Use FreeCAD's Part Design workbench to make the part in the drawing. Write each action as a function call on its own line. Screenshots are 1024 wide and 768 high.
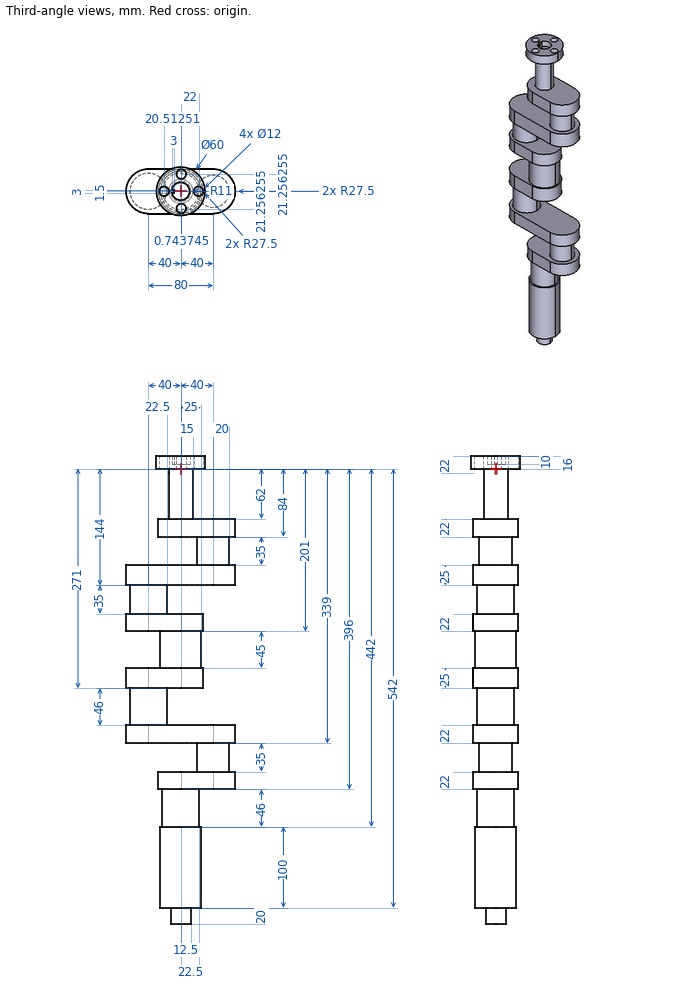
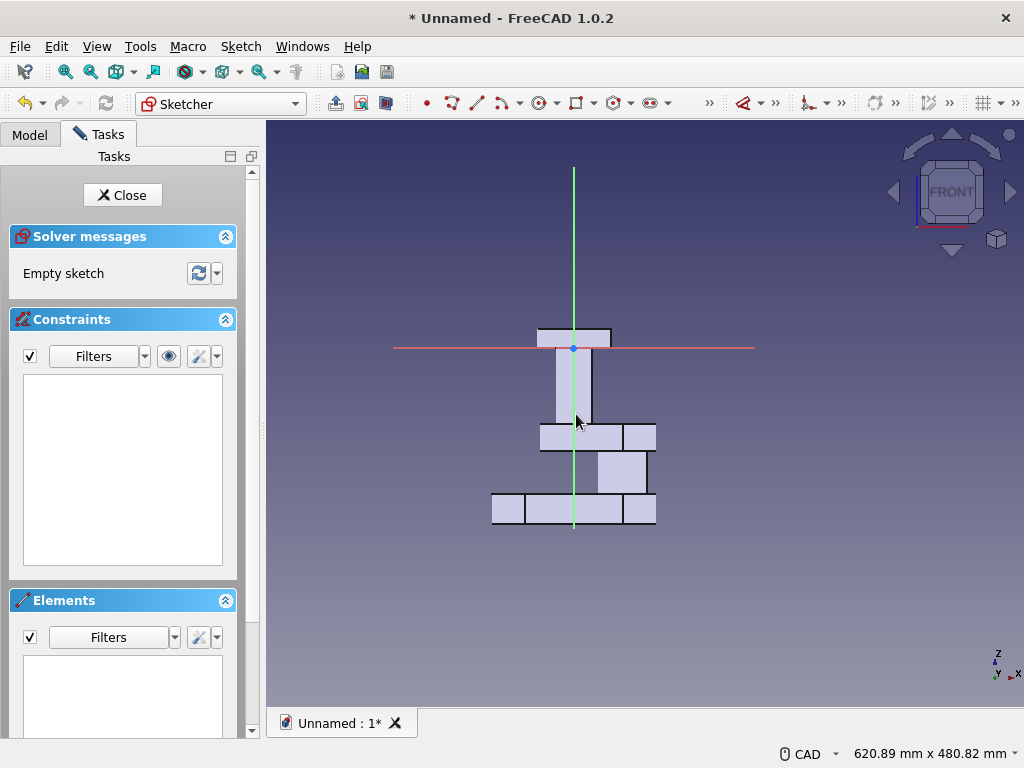
scroll(531, 582, up, 9)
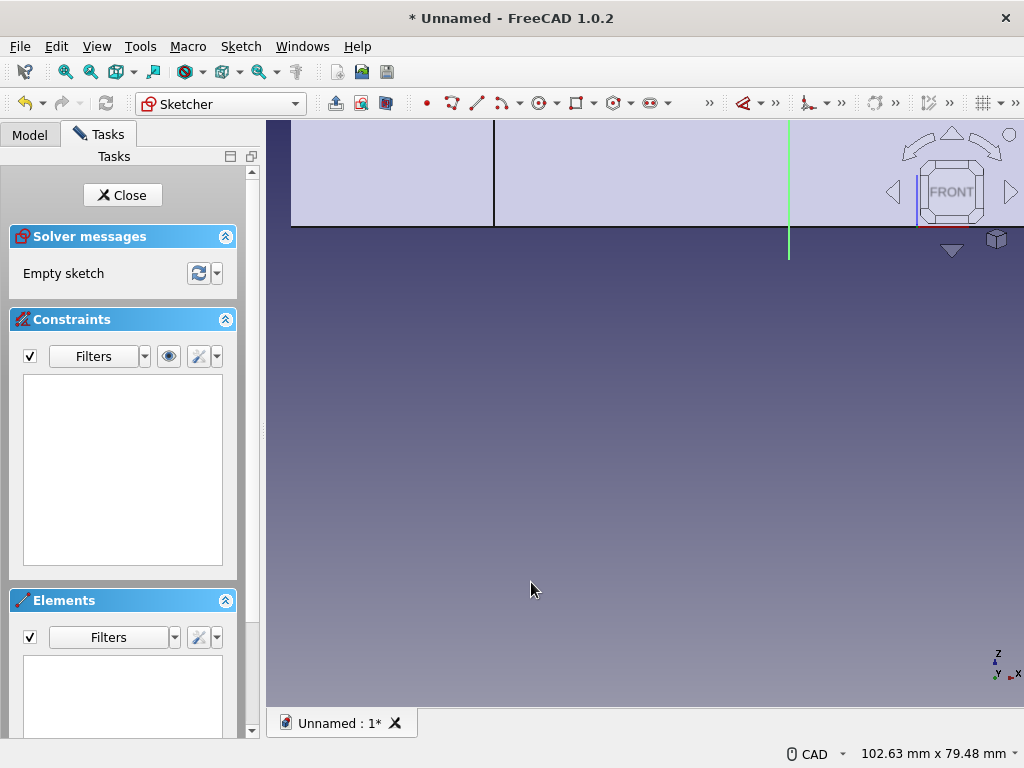
click(576, 104)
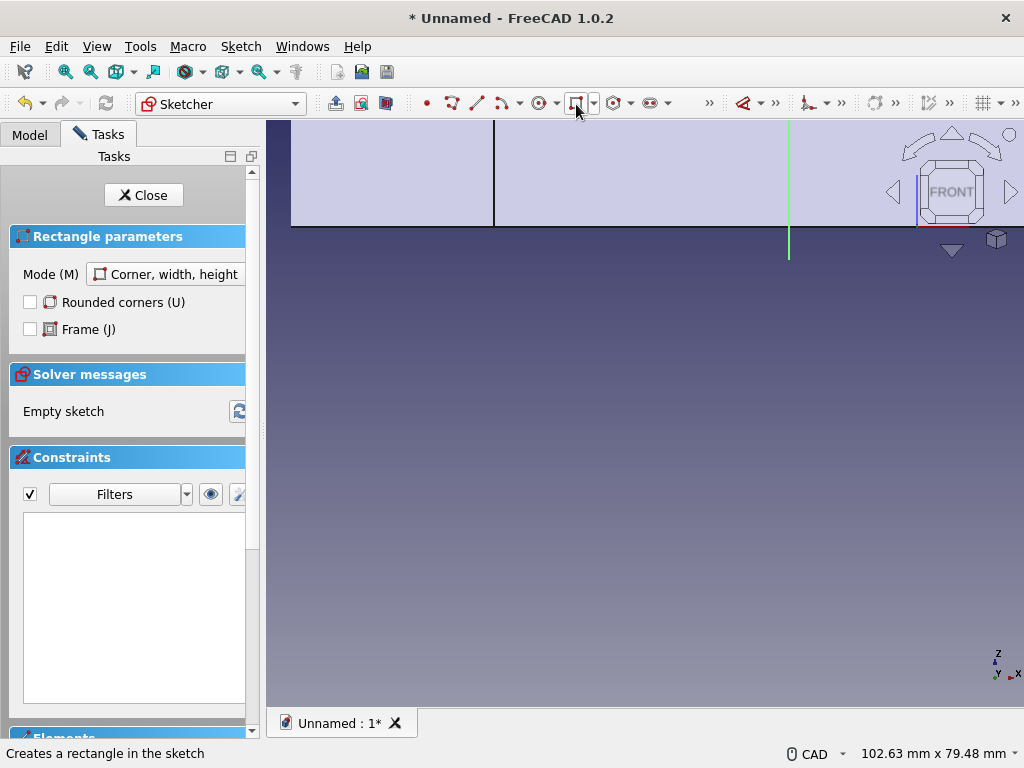
click(494, 227)
move(660, 486)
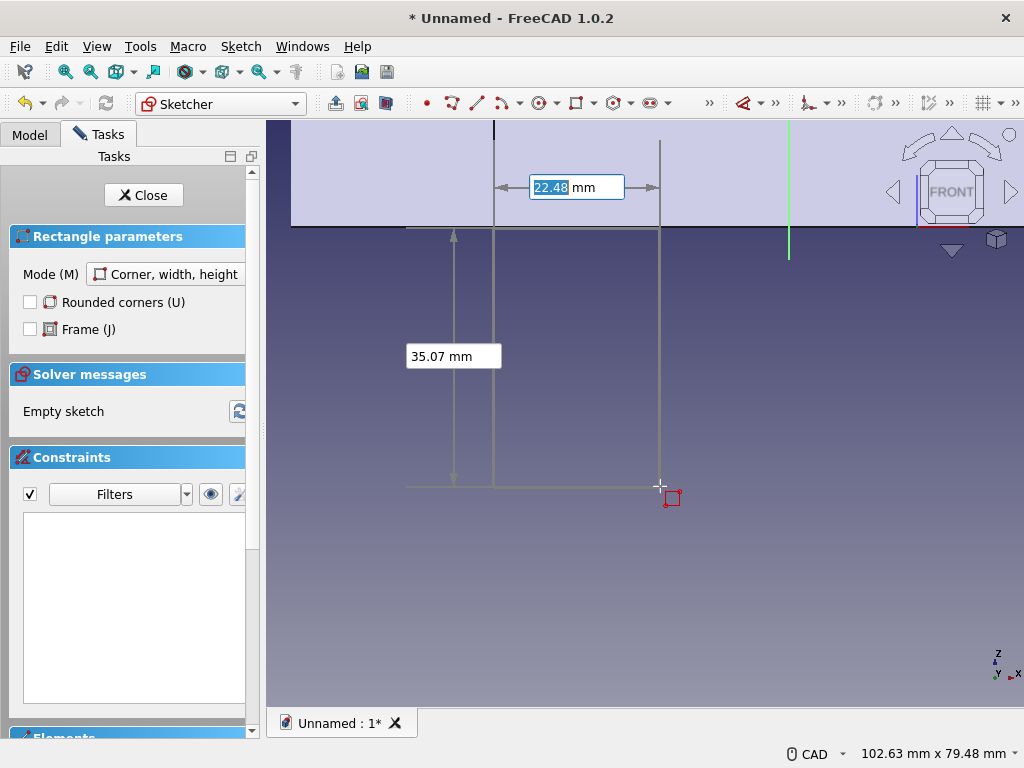
text(22.5)
key(Tab)
text(35)
key(Return)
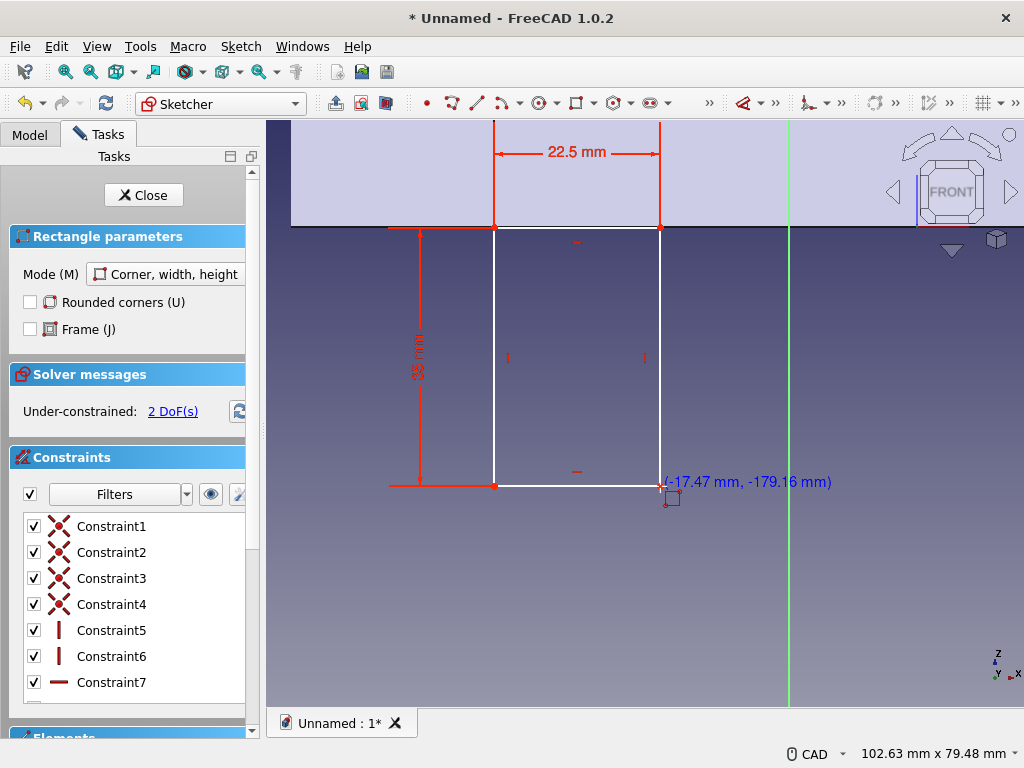
key(g)
key(l)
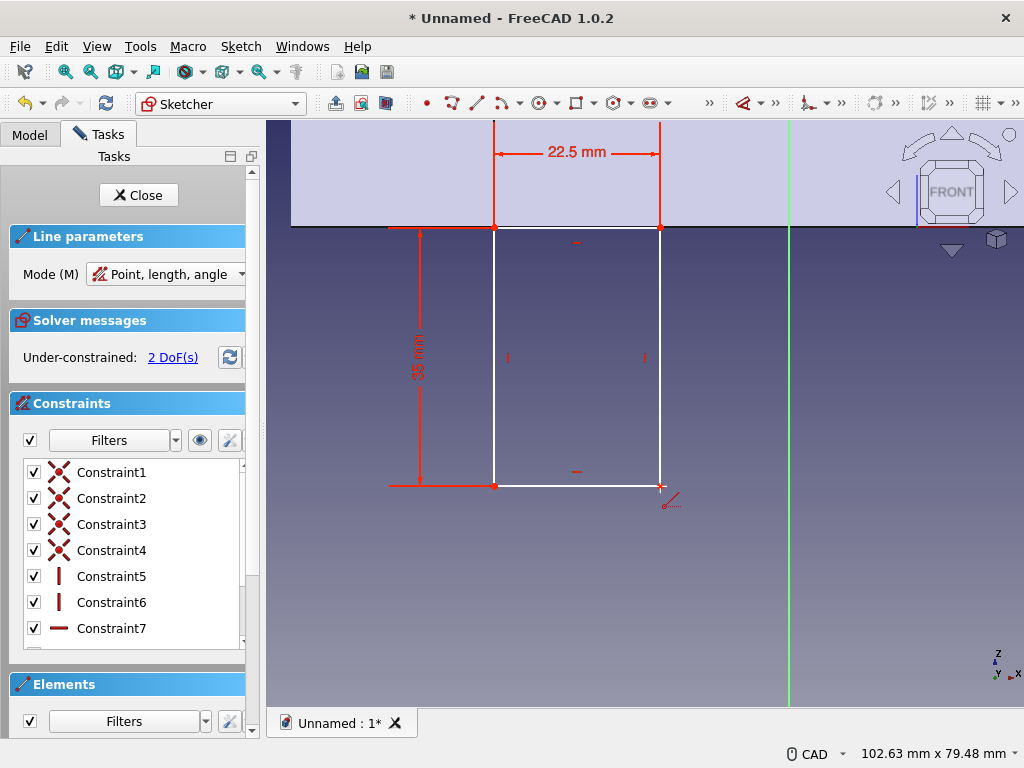
click(494, 512)
click(494, 589)
key(Escape)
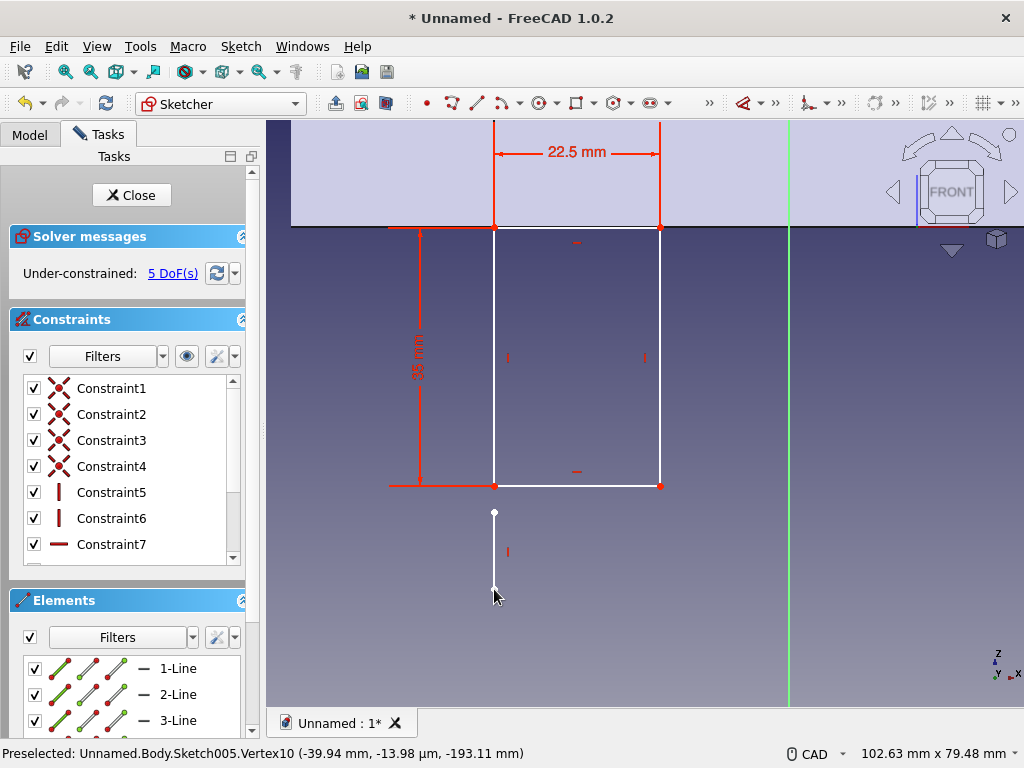
click(494, 536)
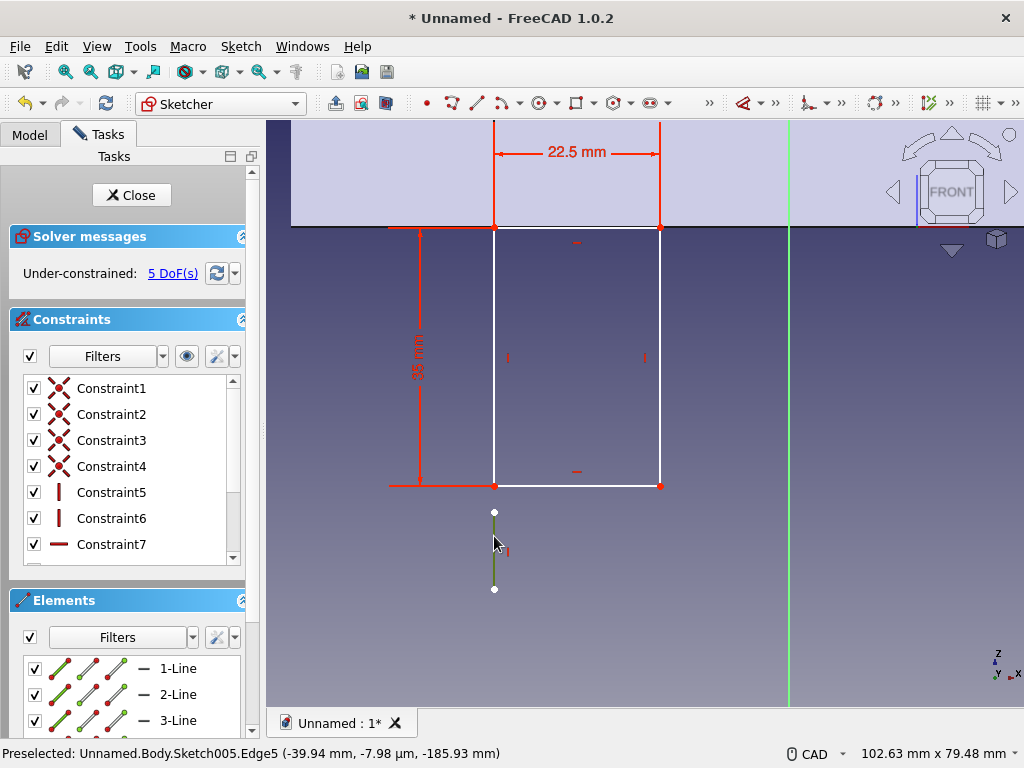
key(g)
key(n)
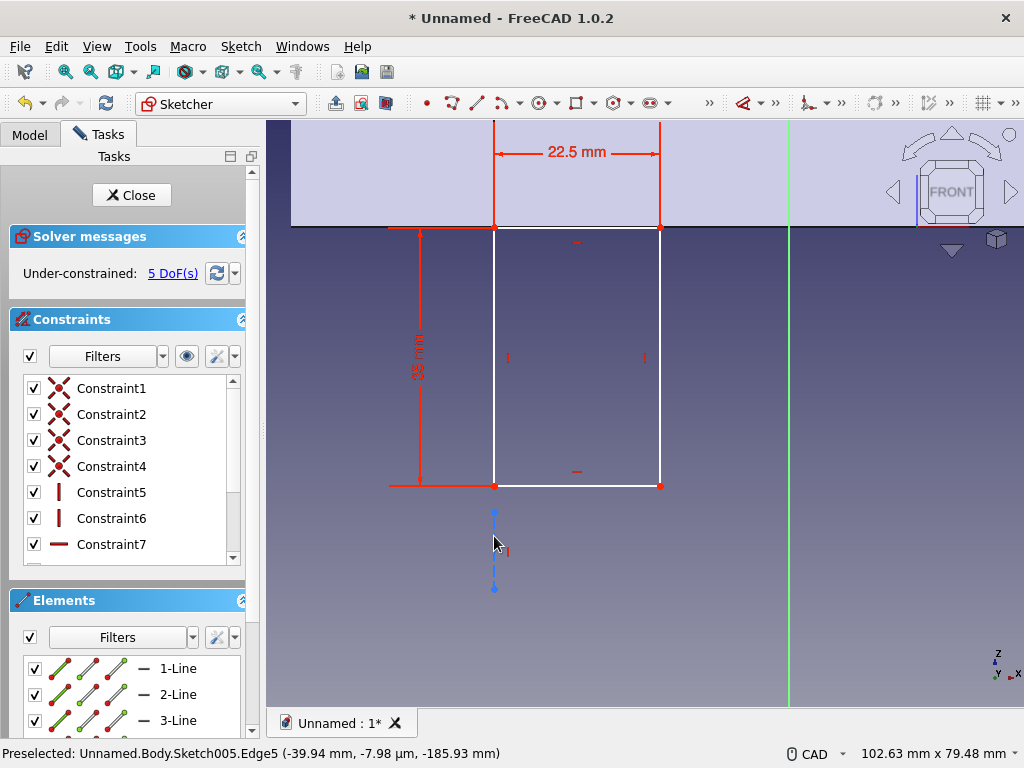
key(d)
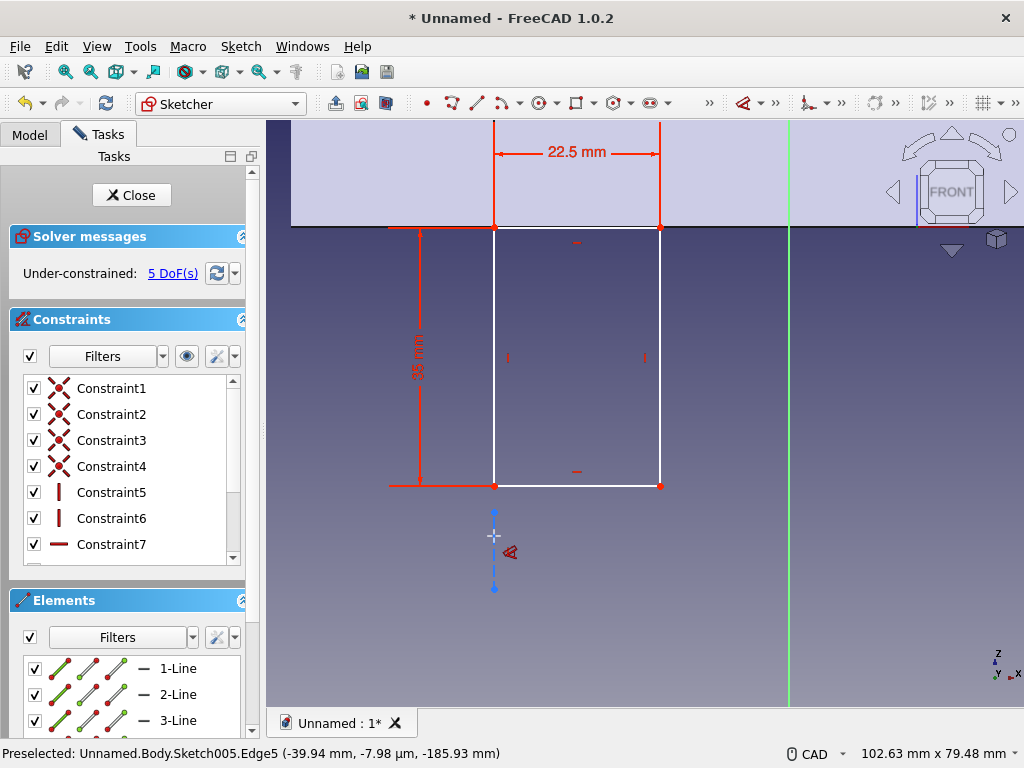
click(494, 228)
click(642, 262)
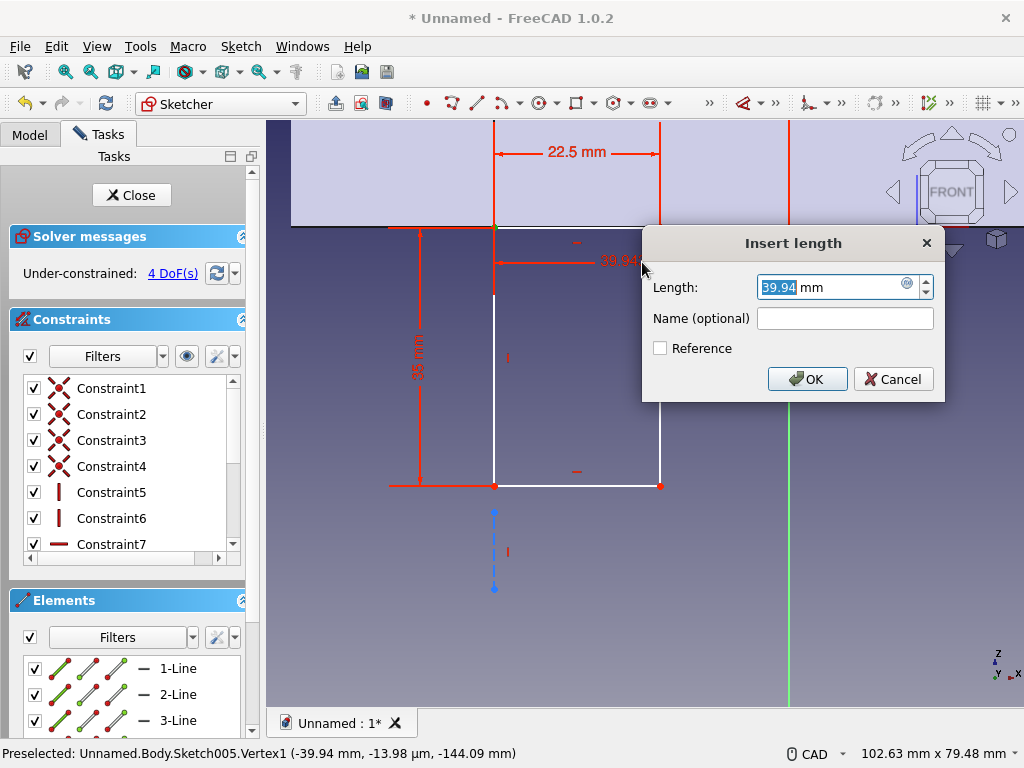
text(40)
key(Return)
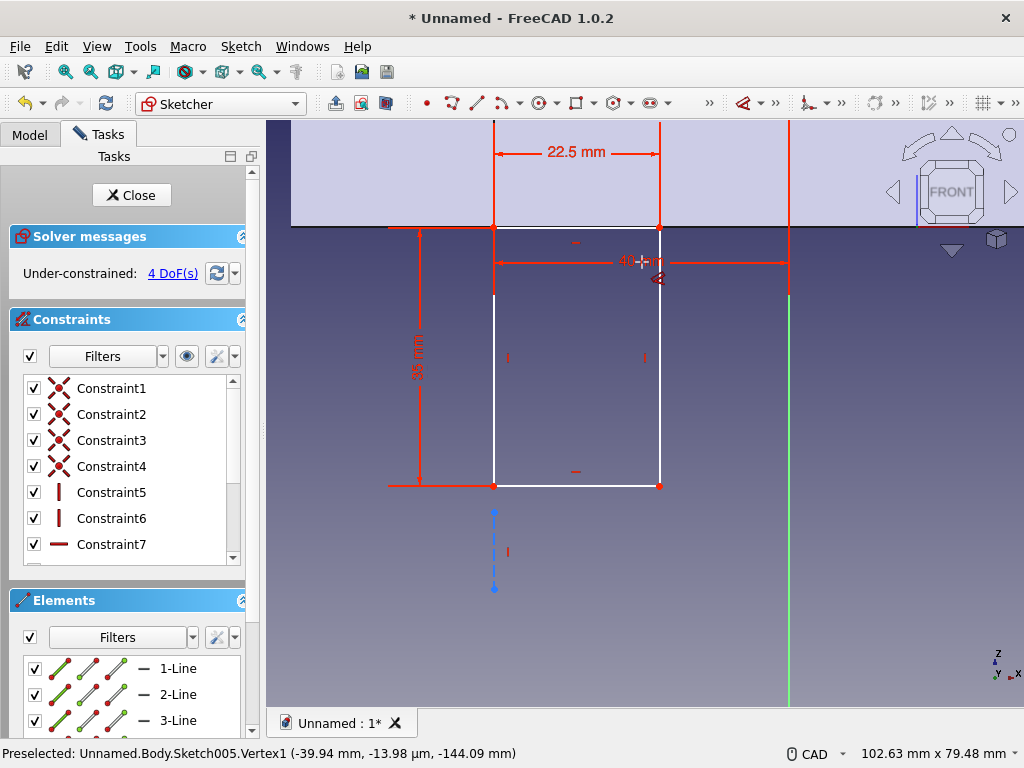
click(494, 513)
click(642, 547)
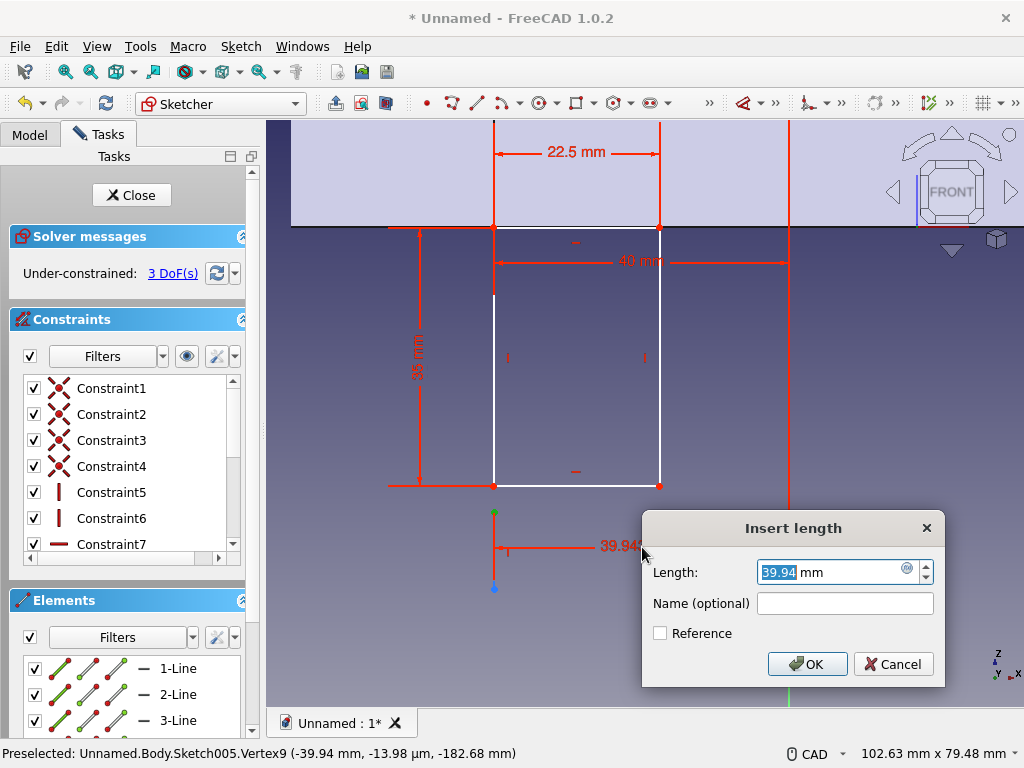
text(40)
key(Return)